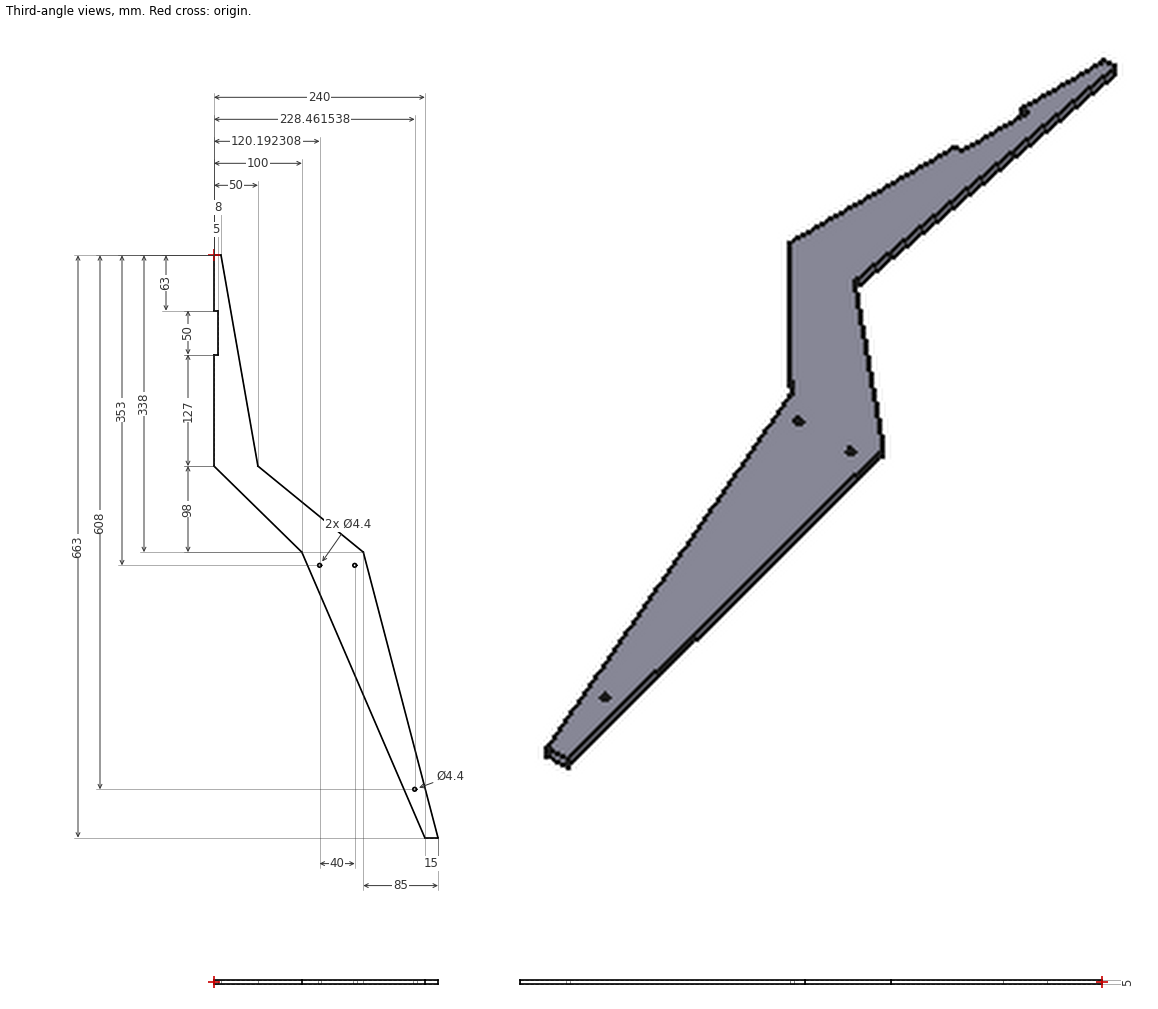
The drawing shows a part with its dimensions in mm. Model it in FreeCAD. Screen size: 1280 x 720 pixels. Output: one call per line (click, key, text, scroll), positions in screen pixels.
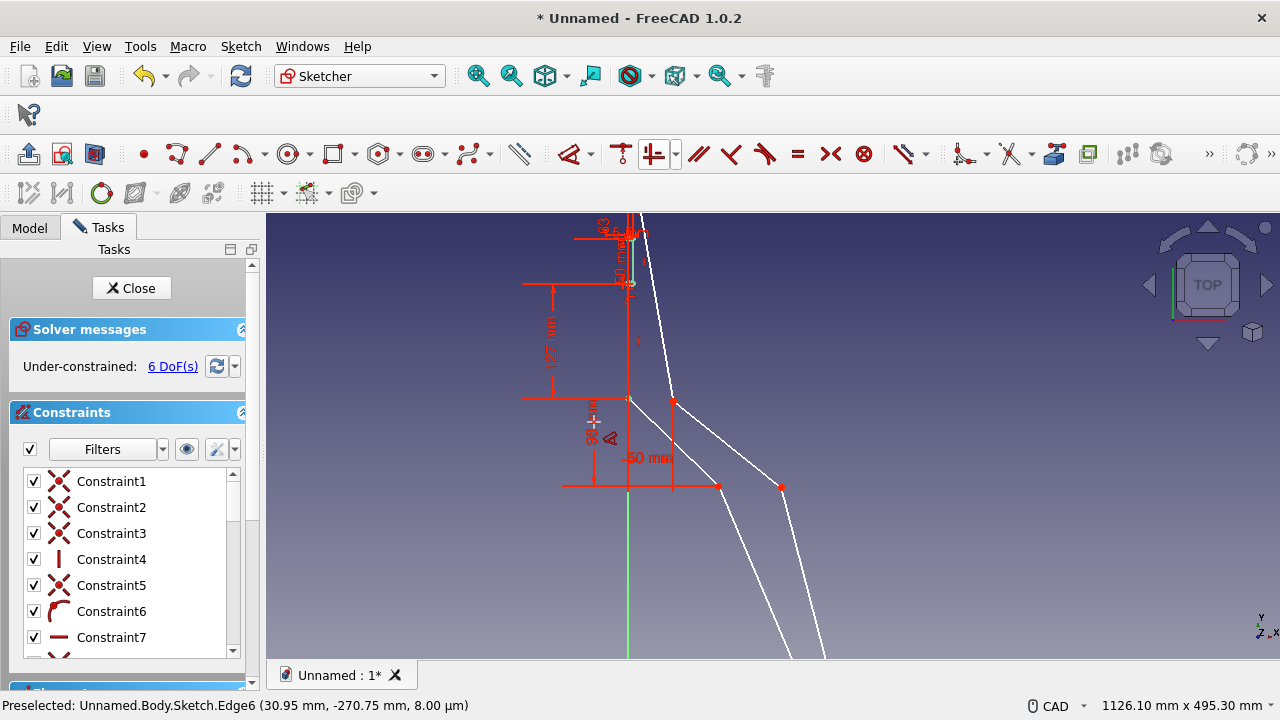
click(804, 576)
click(819, 454)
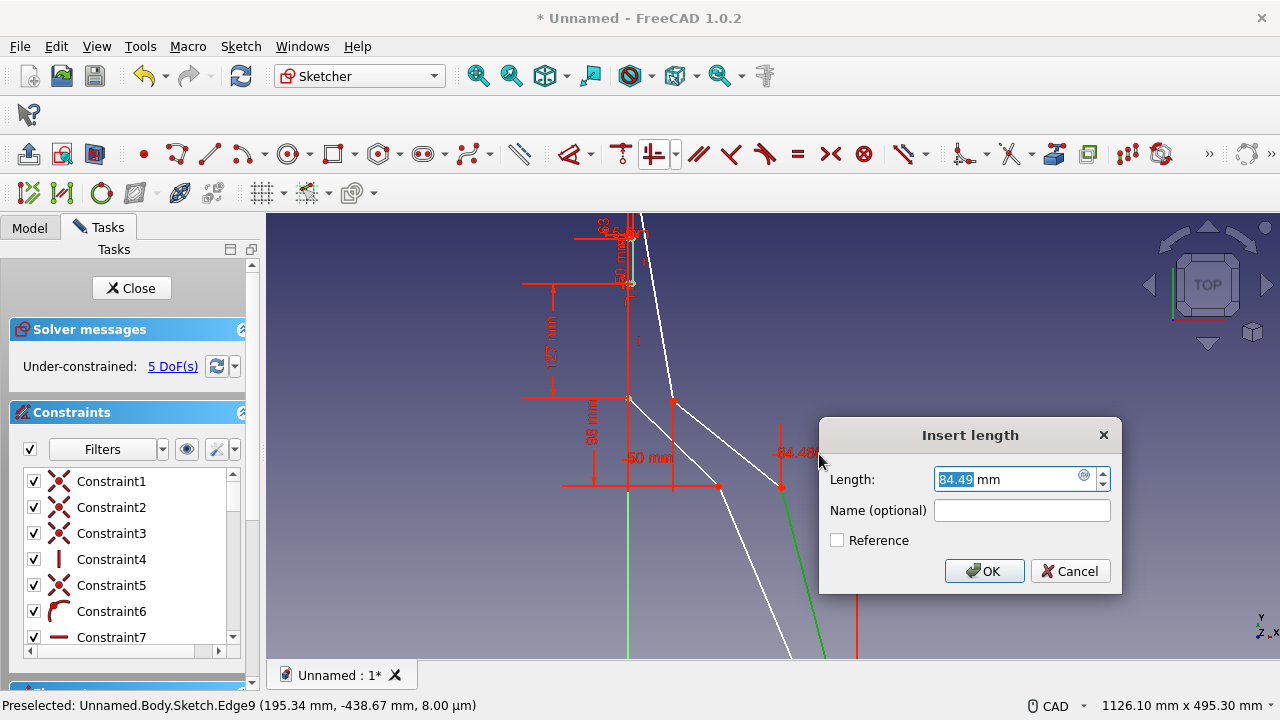
text(85)
key(Return)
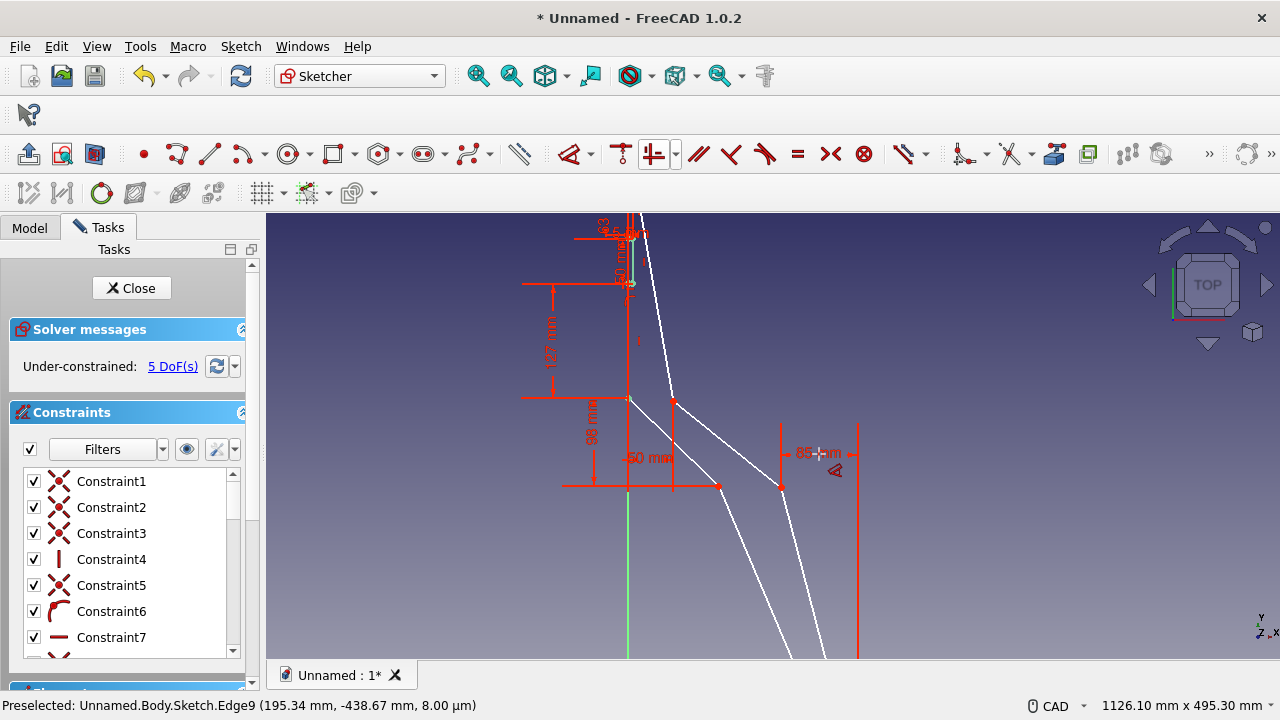
click(749, 462)
click(815, 425)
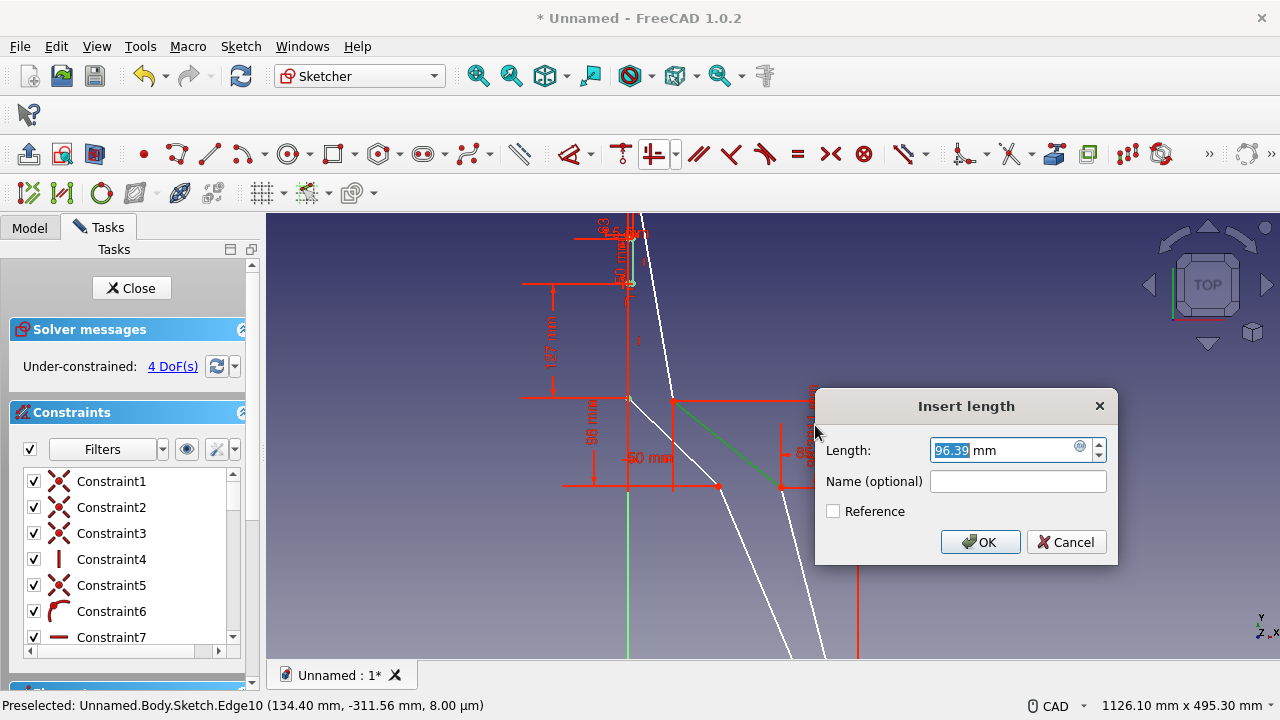
text(98)
key(Return)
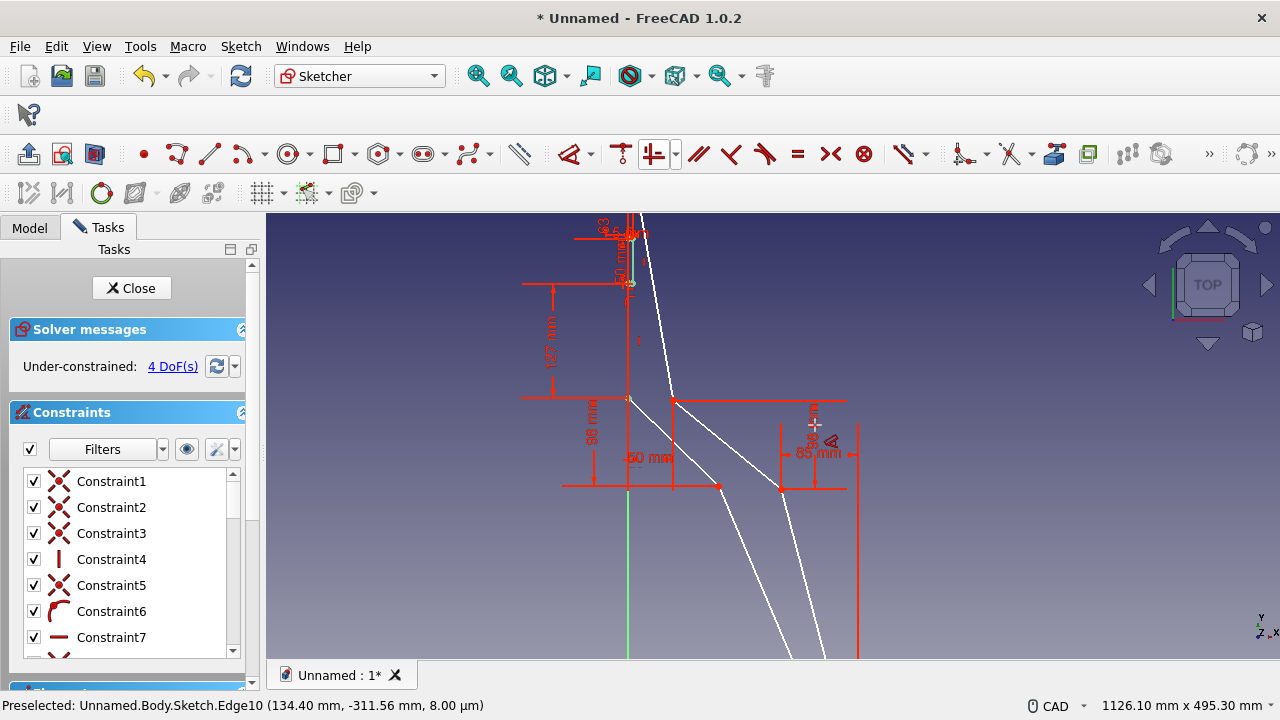
click(719, 486)
click(674, 520)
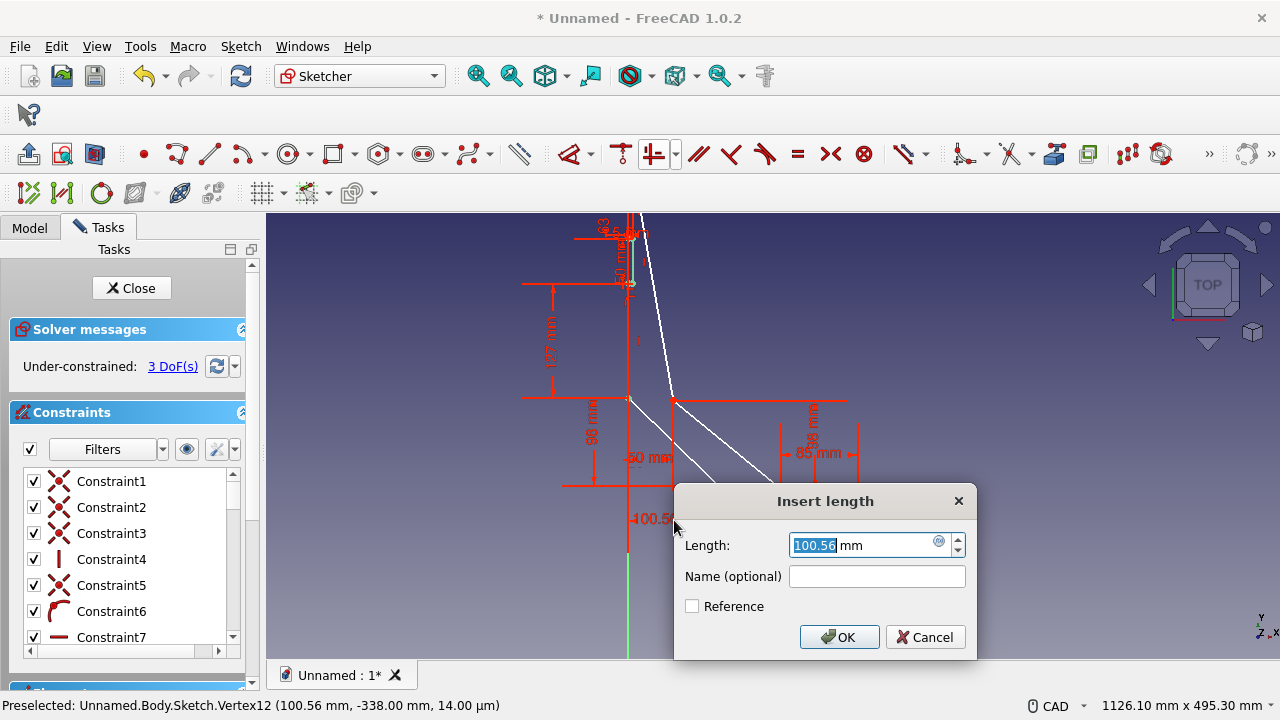
text(100)
key(Return)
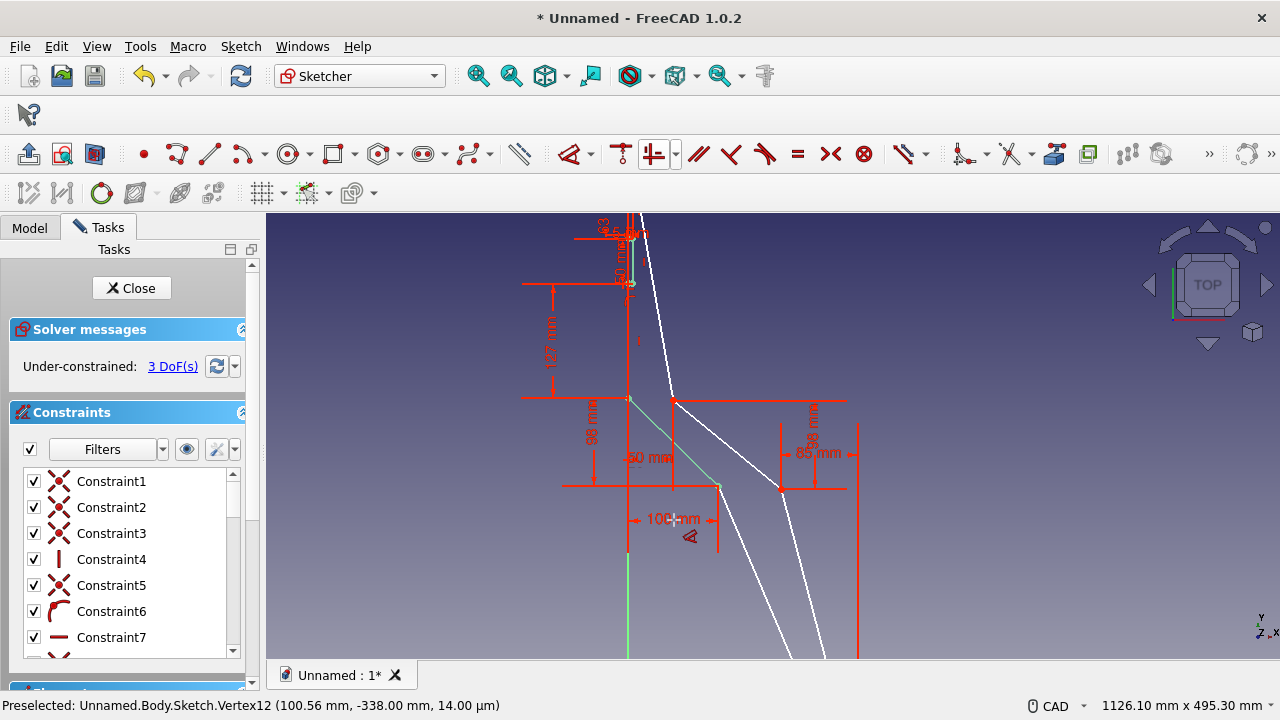
scroll(673, 400, down, 4)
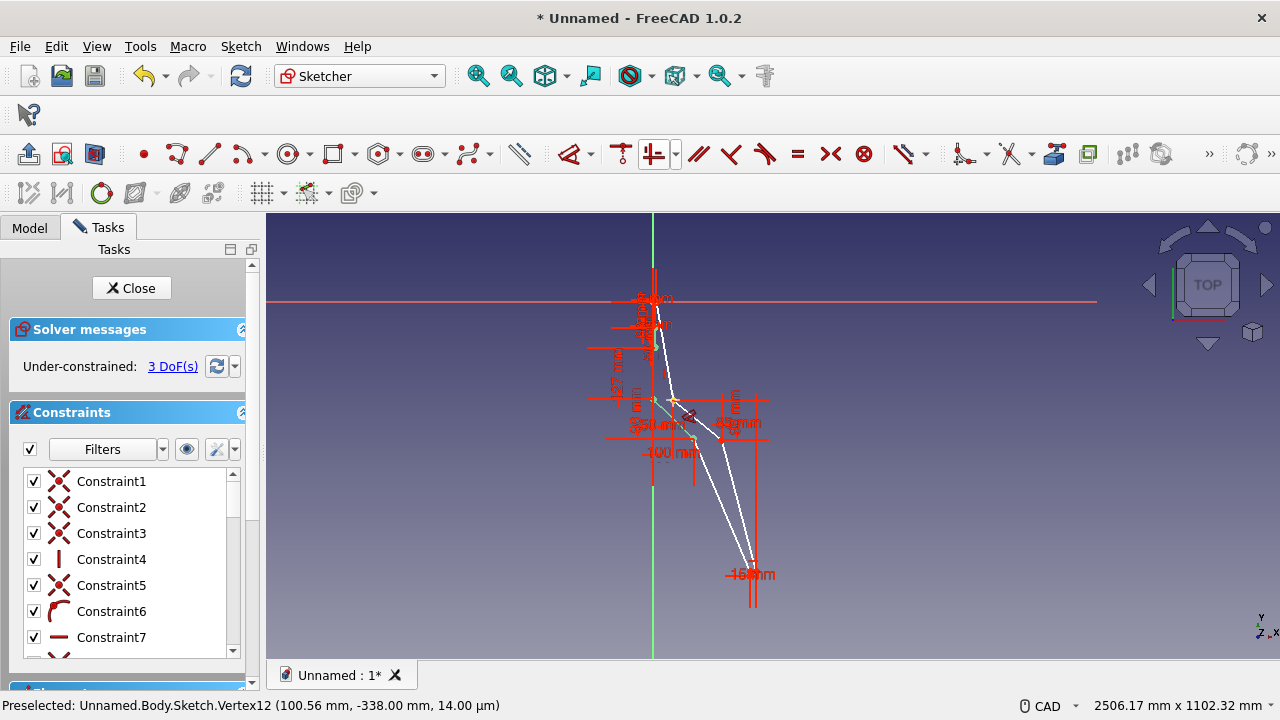
scroll(750, 572, up, 4)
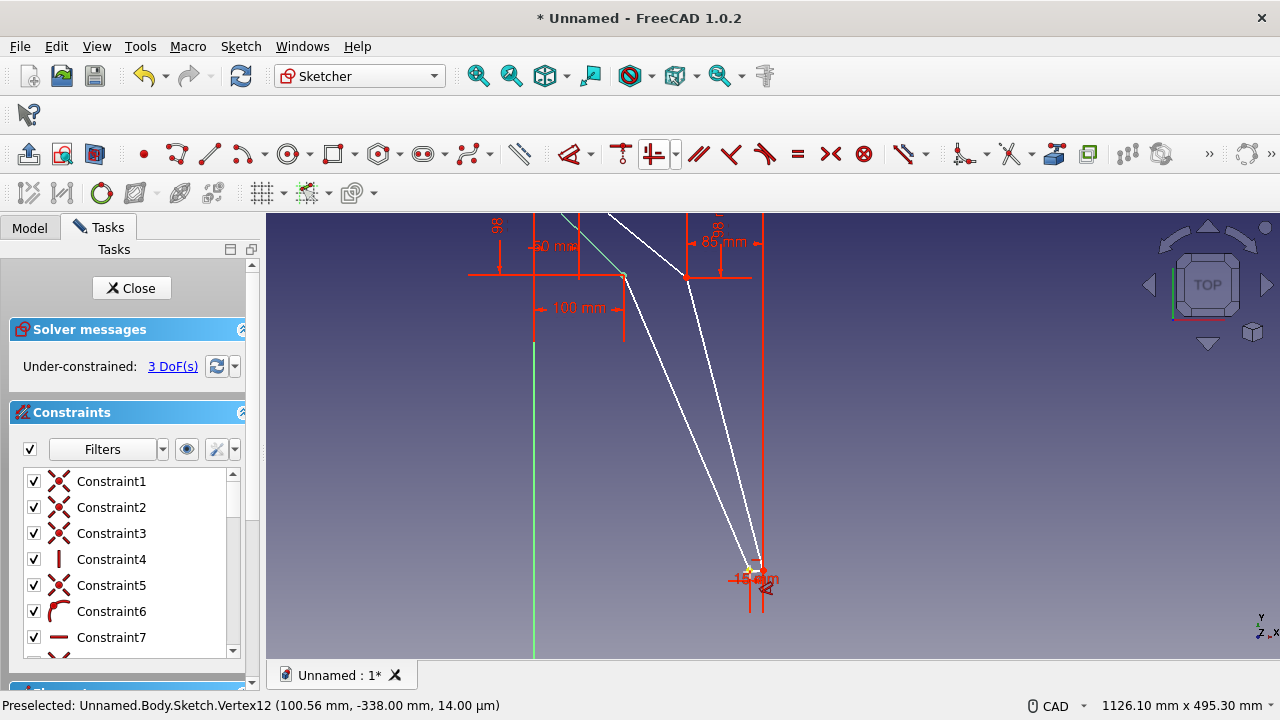
click(750, 571)
click(642, 605)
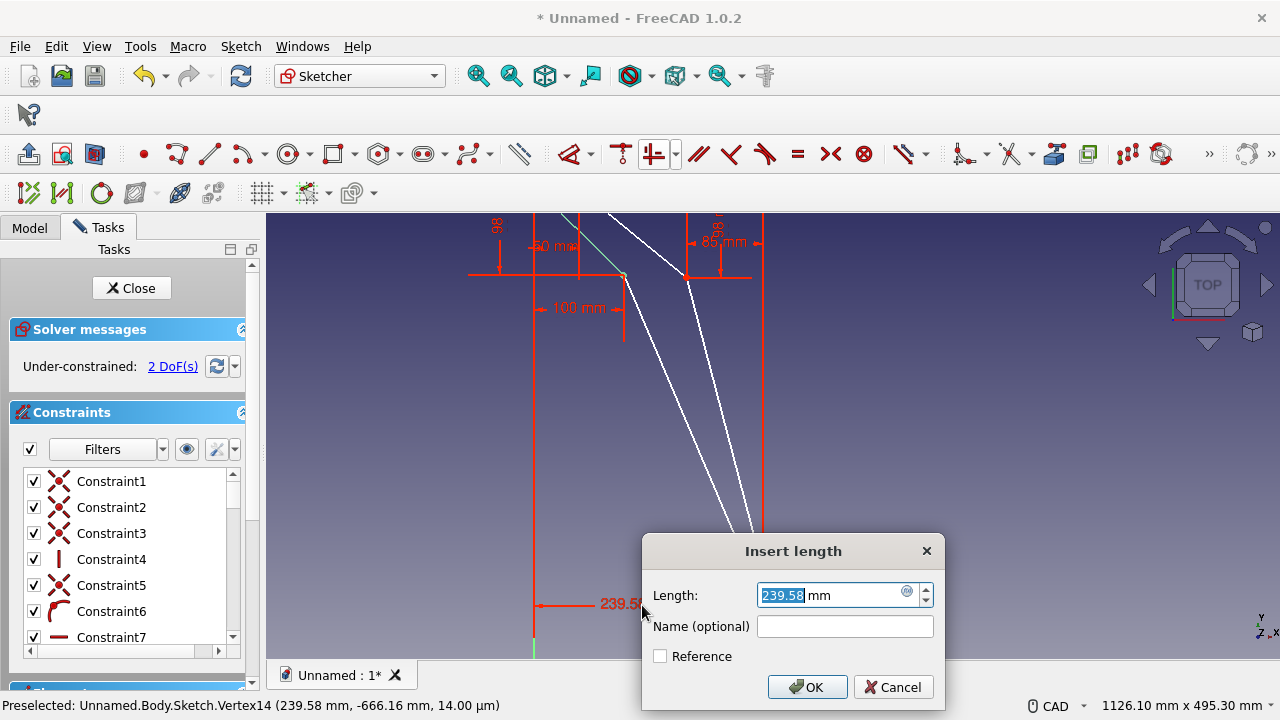
text(240)
key(Return)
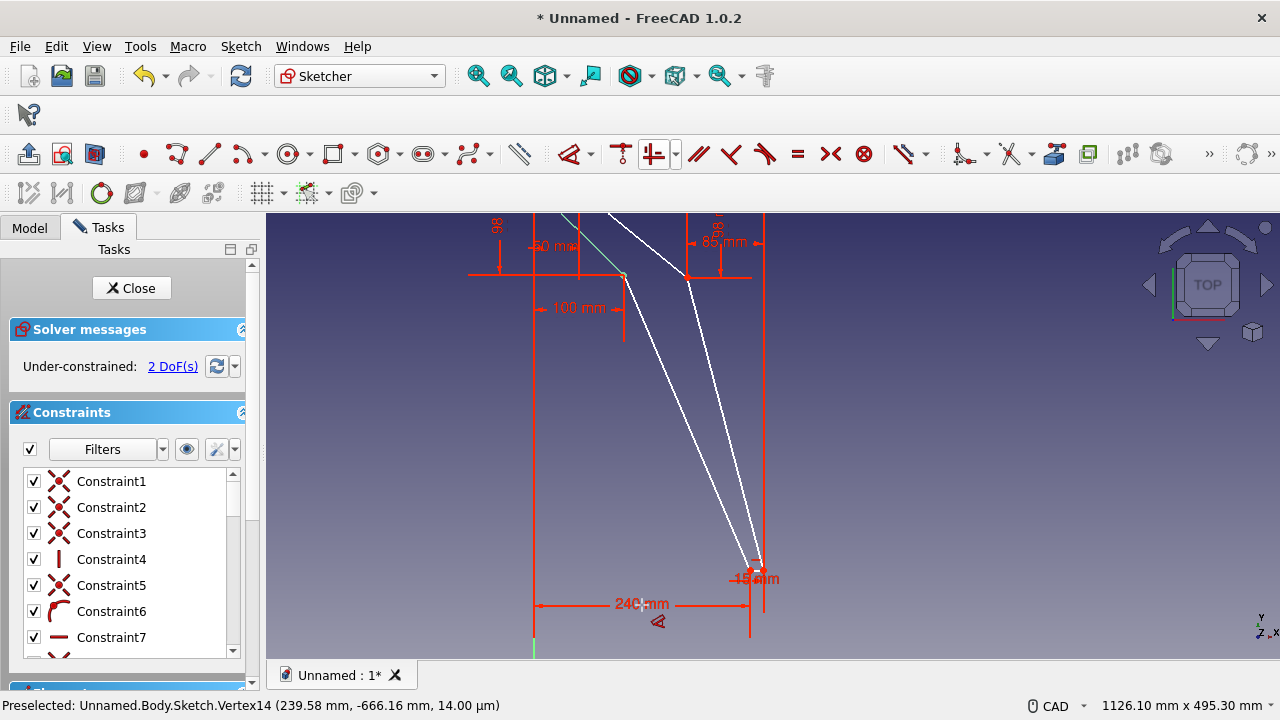
click(750, 571)
click(500, 406)